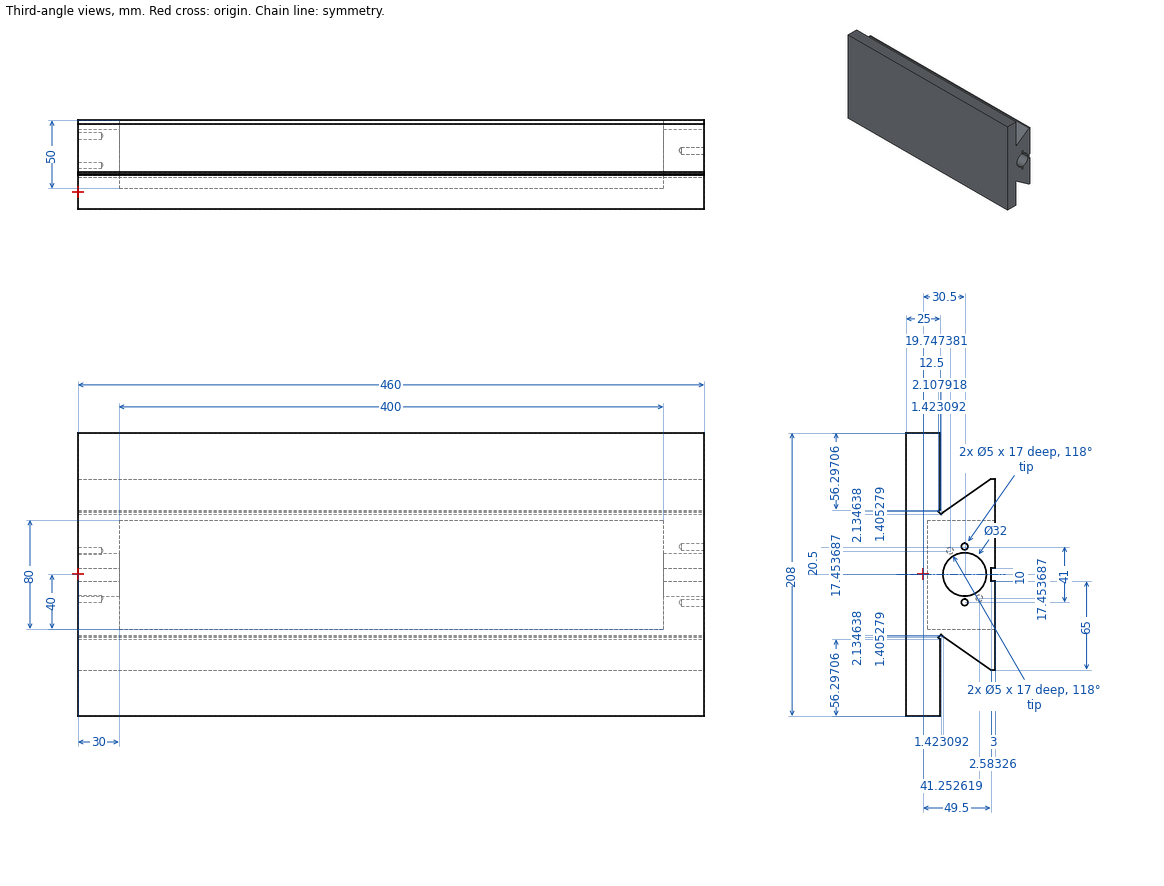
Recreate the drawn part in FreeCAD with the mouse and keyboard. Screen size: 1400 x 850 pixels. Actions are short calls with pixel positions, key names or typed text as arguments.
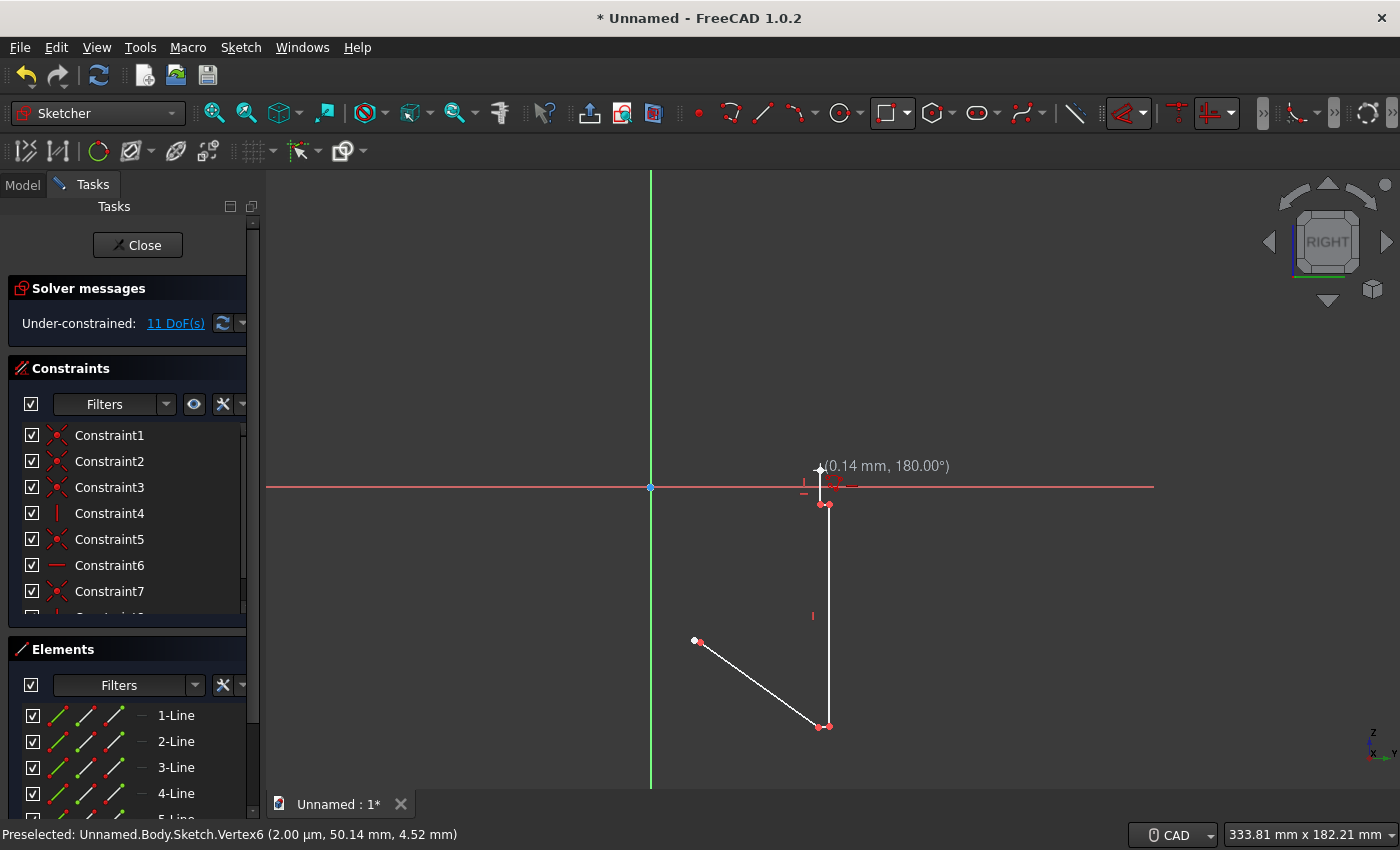
scroll(829, 470, up, 3)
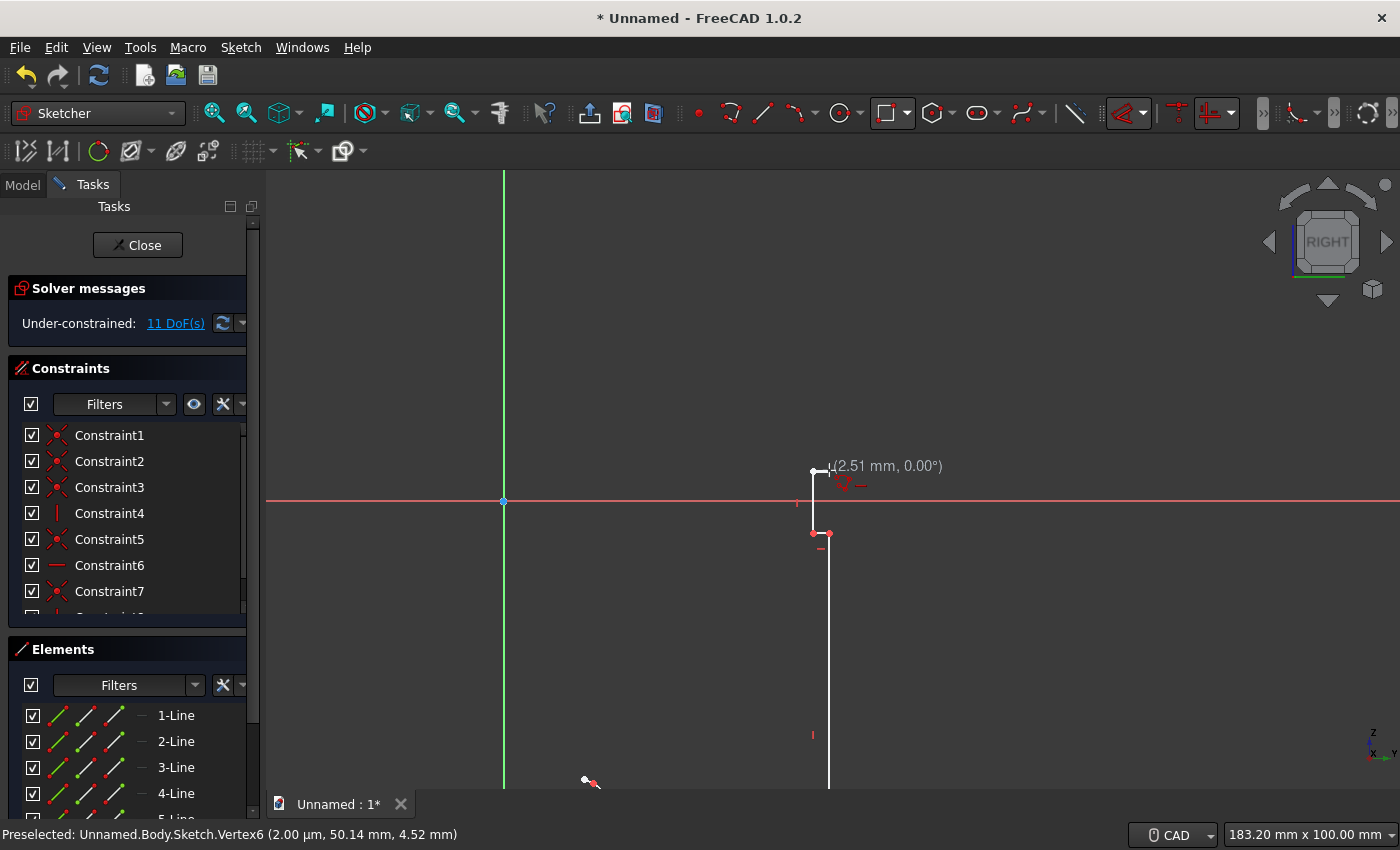
click(829, 470)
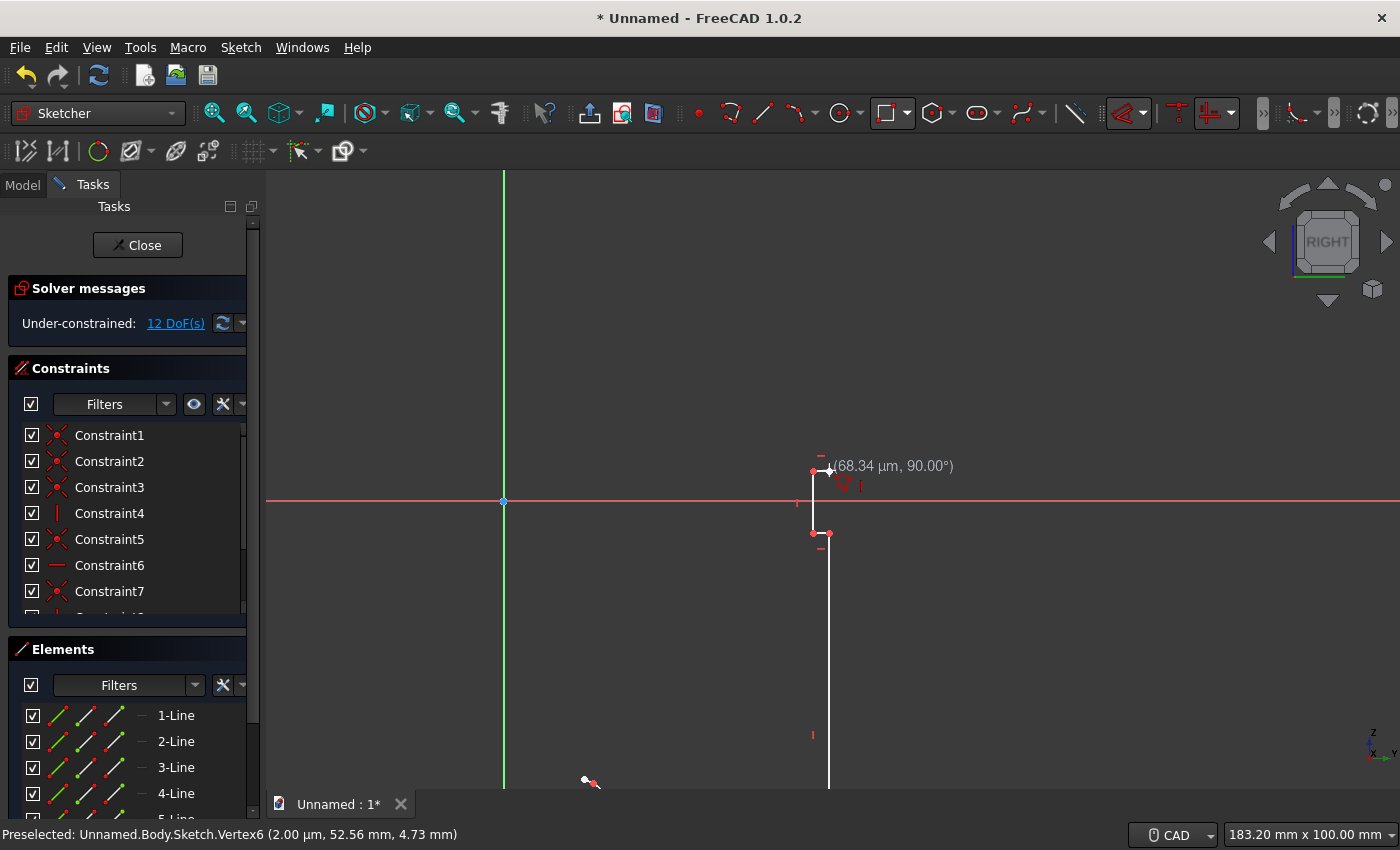
scroll(824, 470, down, 6)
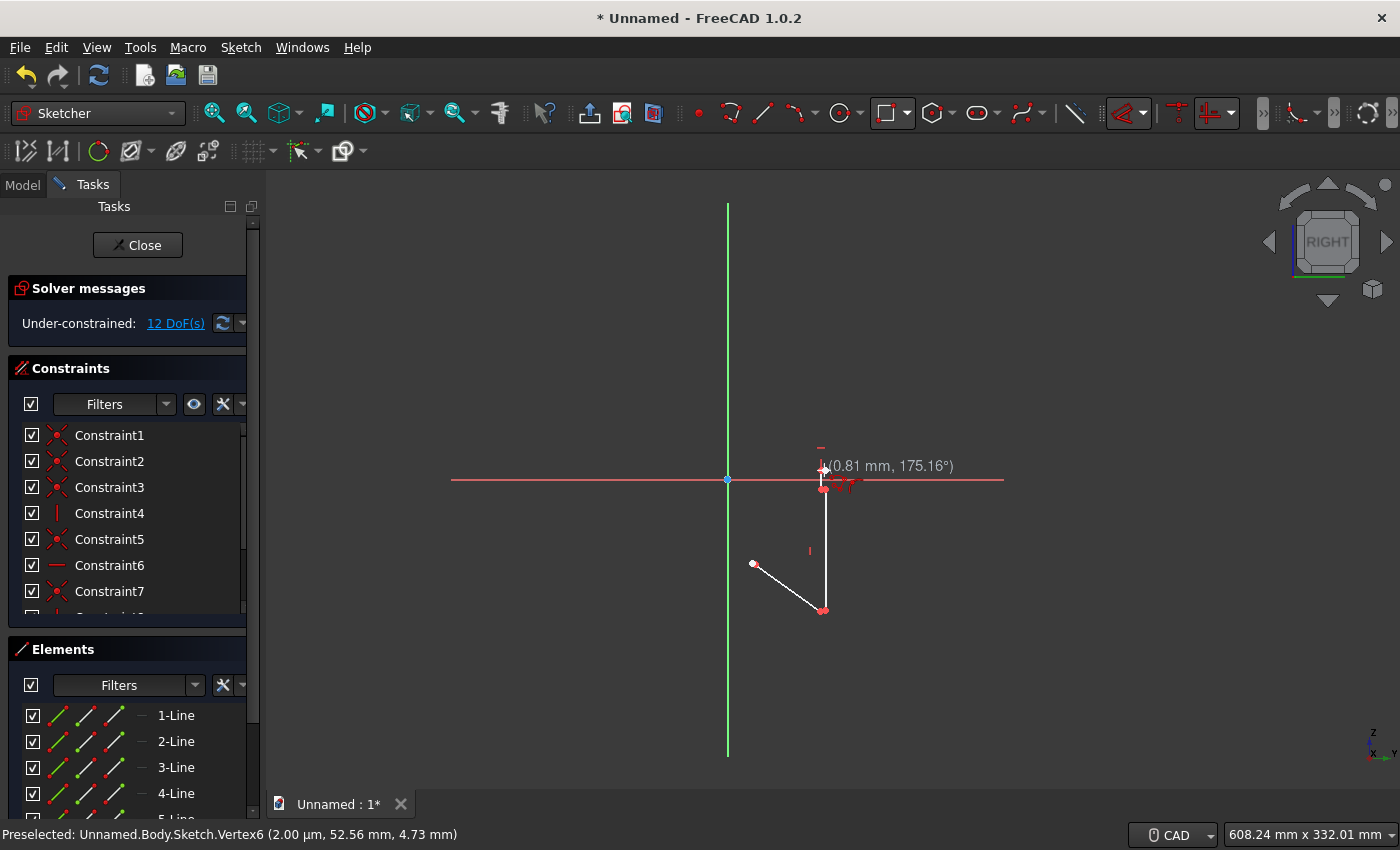
click(826, 349)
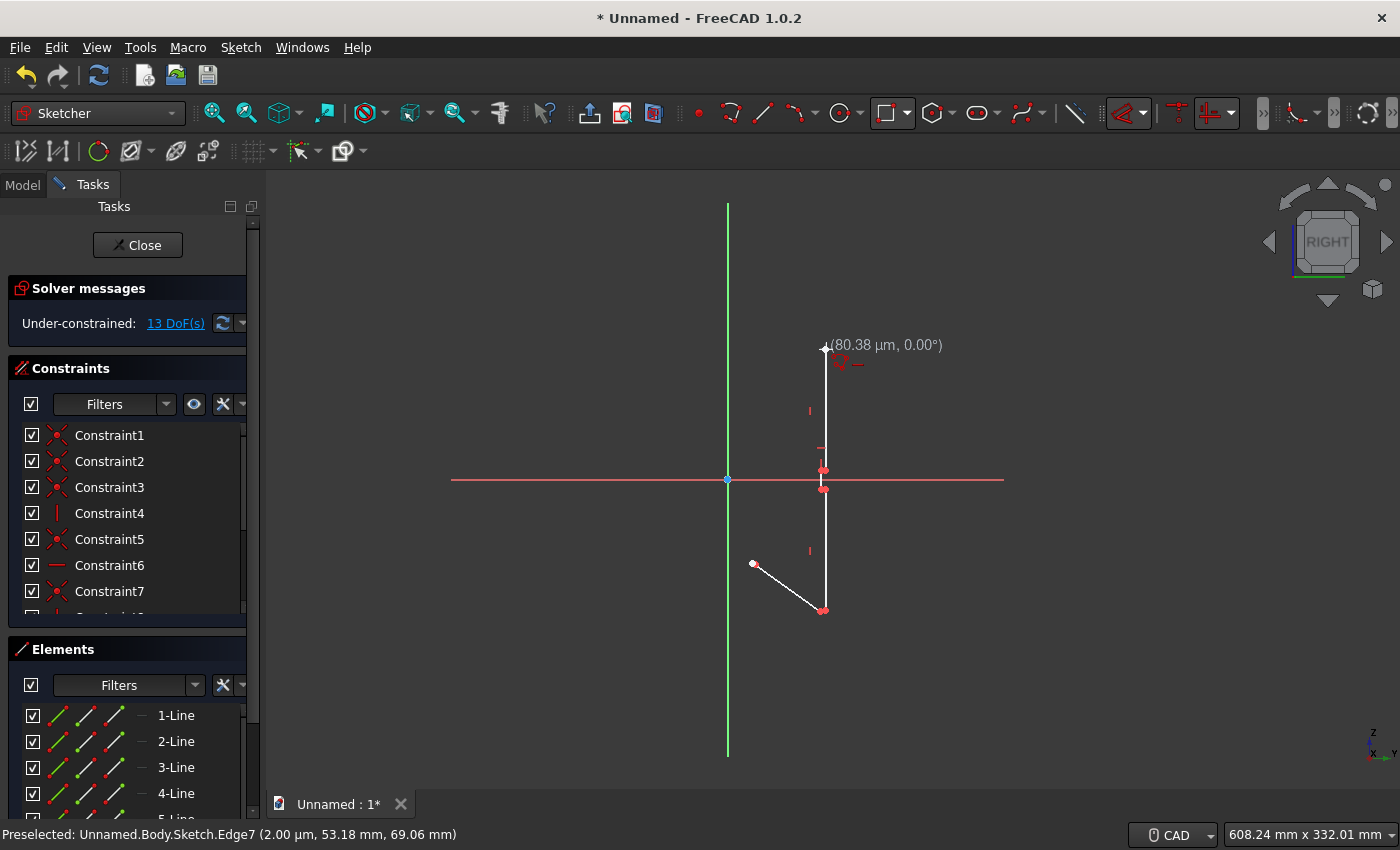
scroll(820, 349, up, 6)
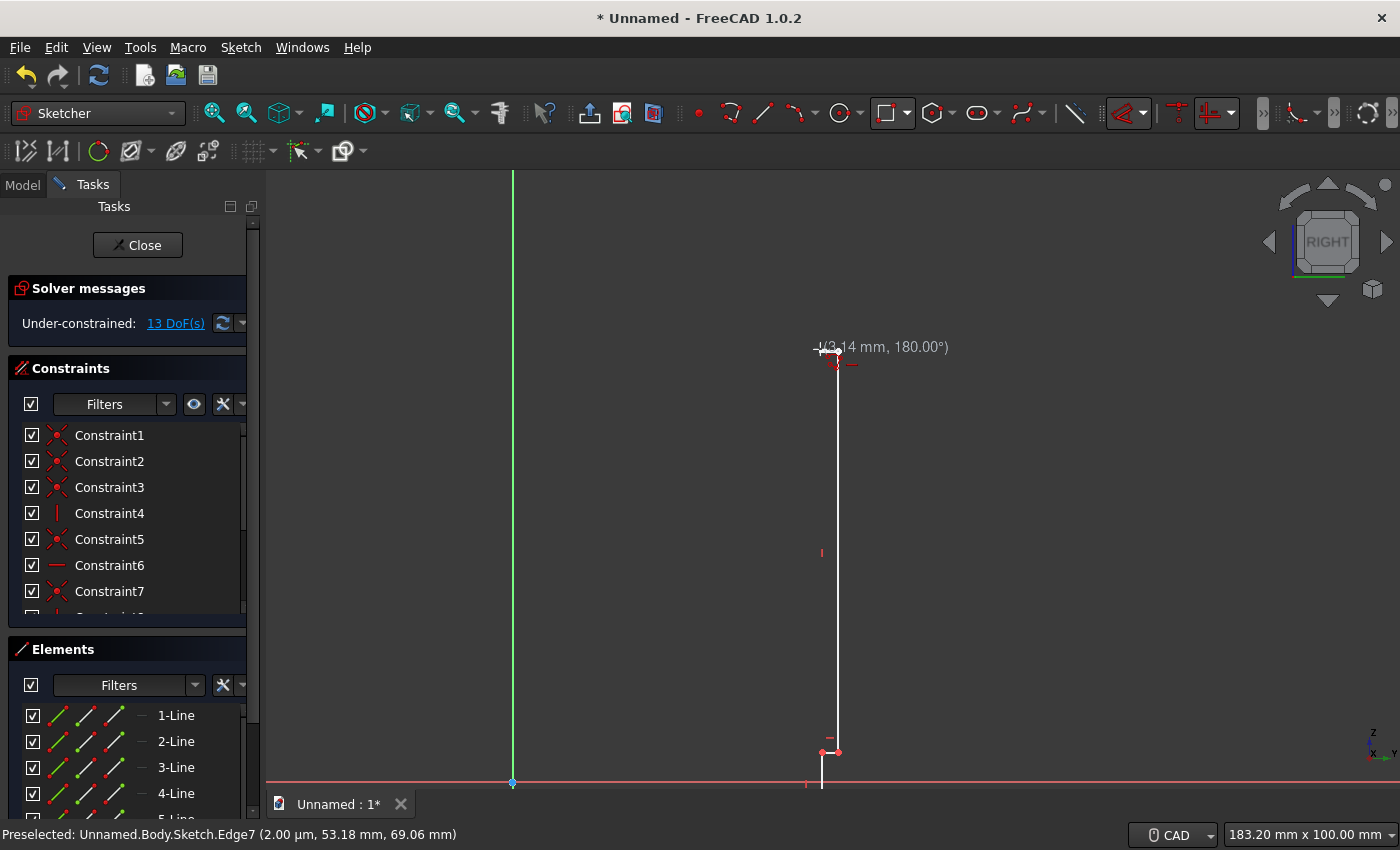
click(819, 348)
click(603, 500)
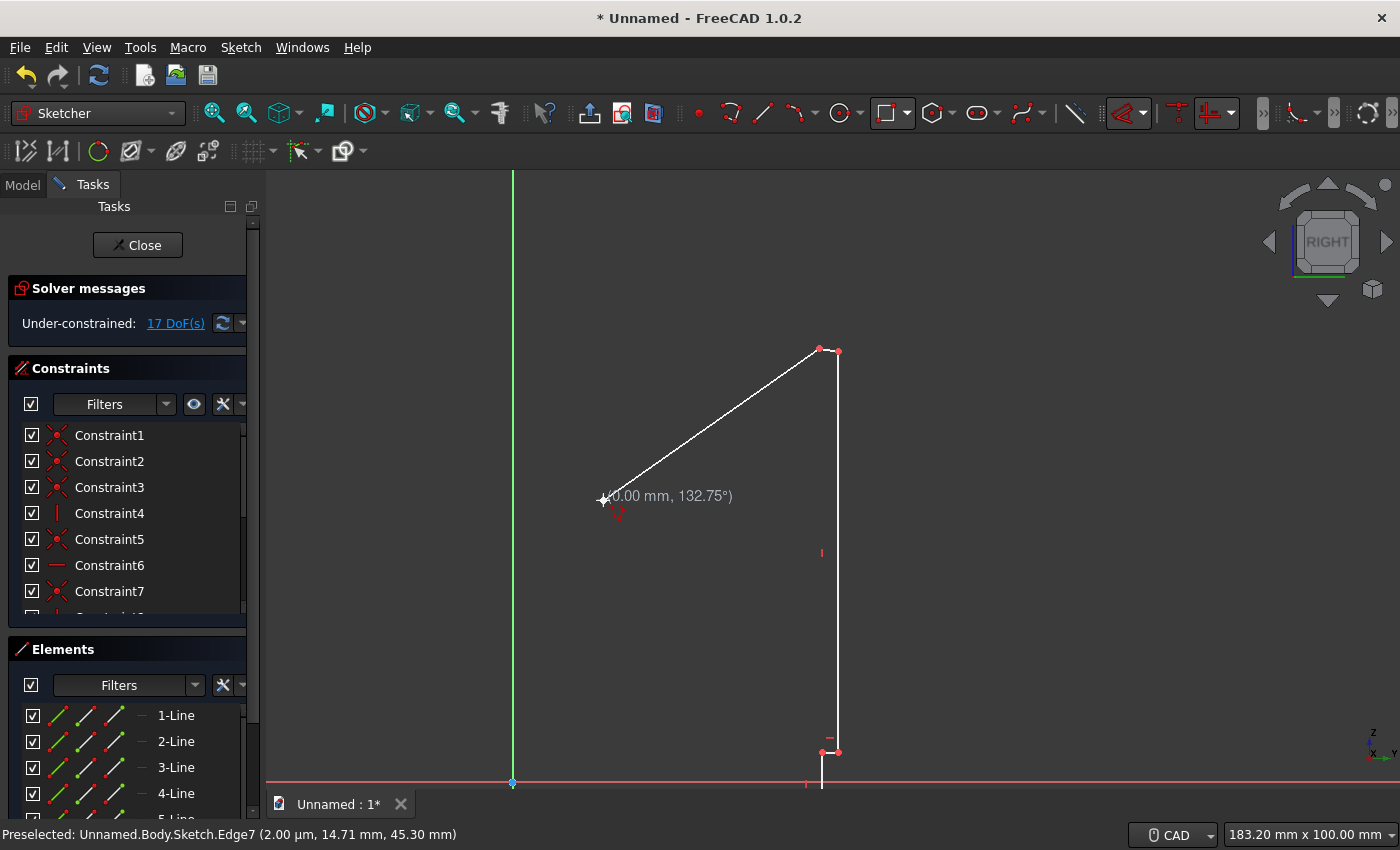
scroll(595, 509, up, 2)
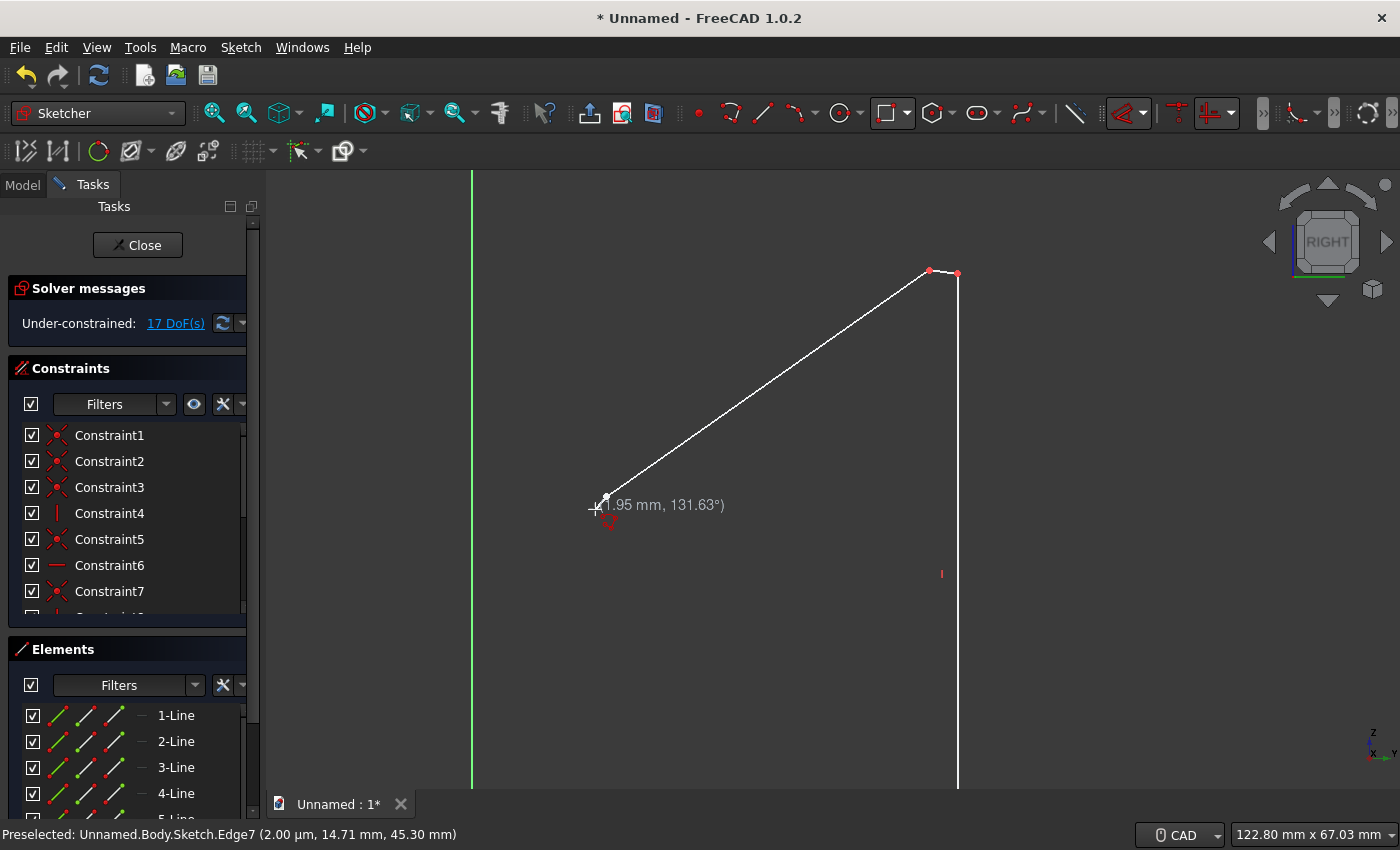
click(594, 509)
click(575, 489)
click(588, 476)